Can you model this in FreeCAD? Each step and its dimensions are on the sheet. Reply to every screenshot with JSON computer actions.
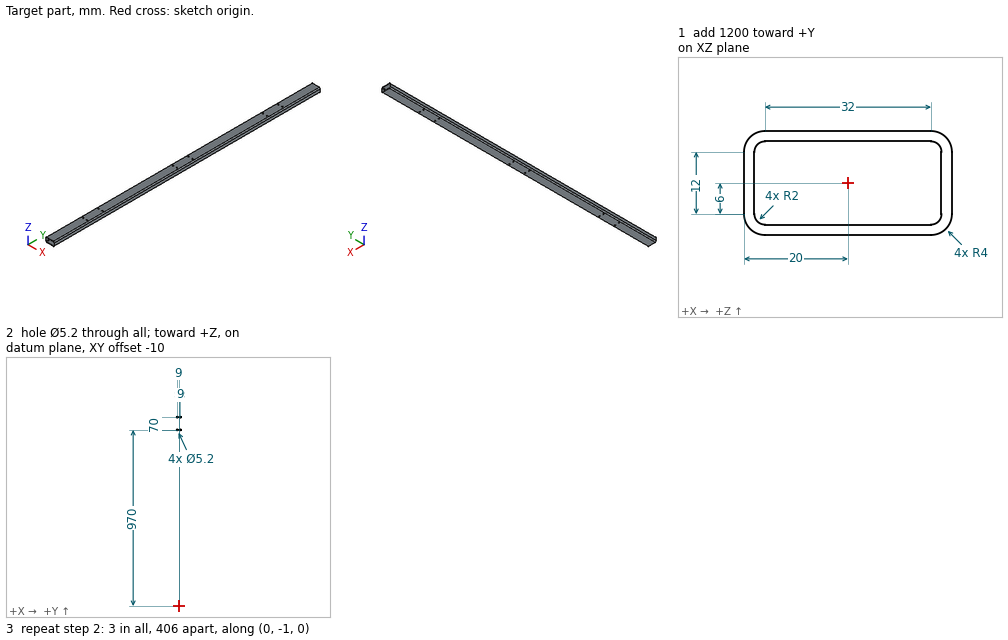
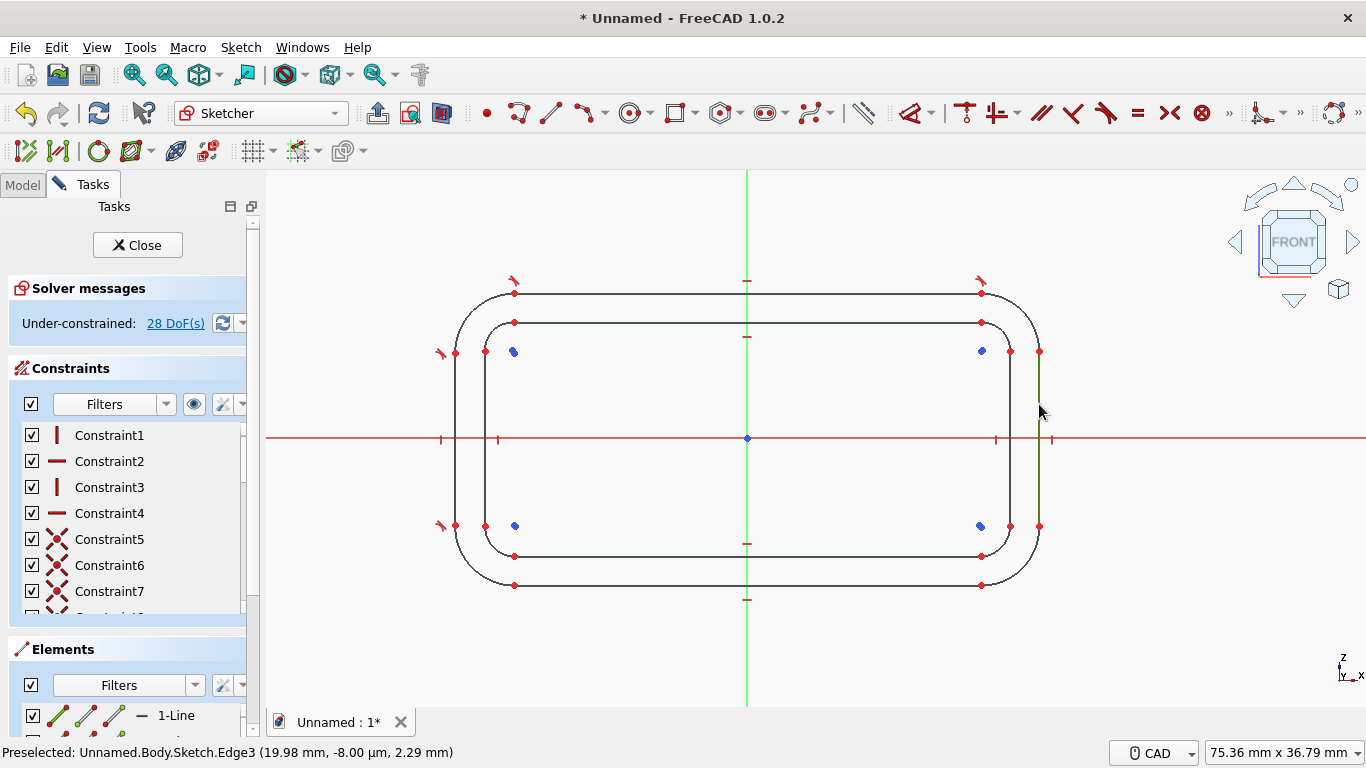
{"action": "left_click", "coordinate": [1033, 325]}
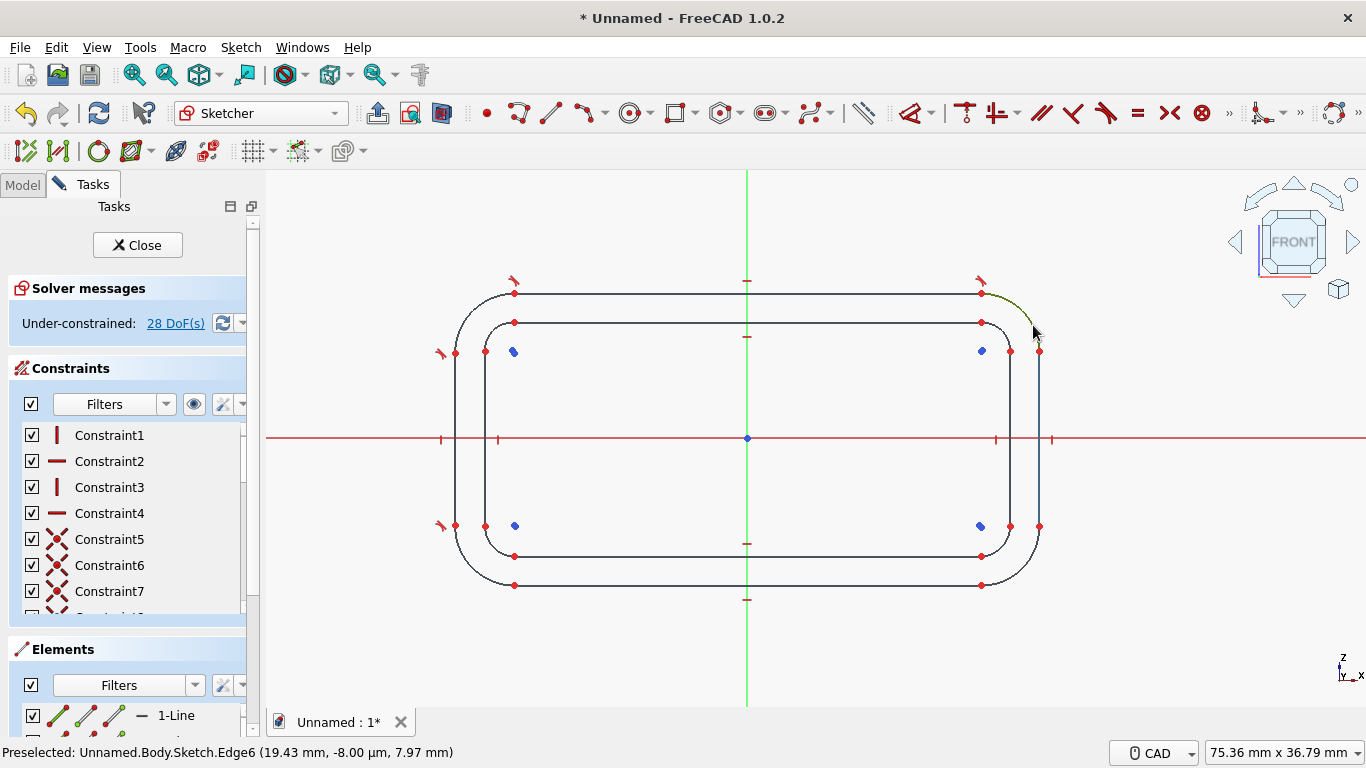
{"action": "left_click", "coordinate": [1106, 114]}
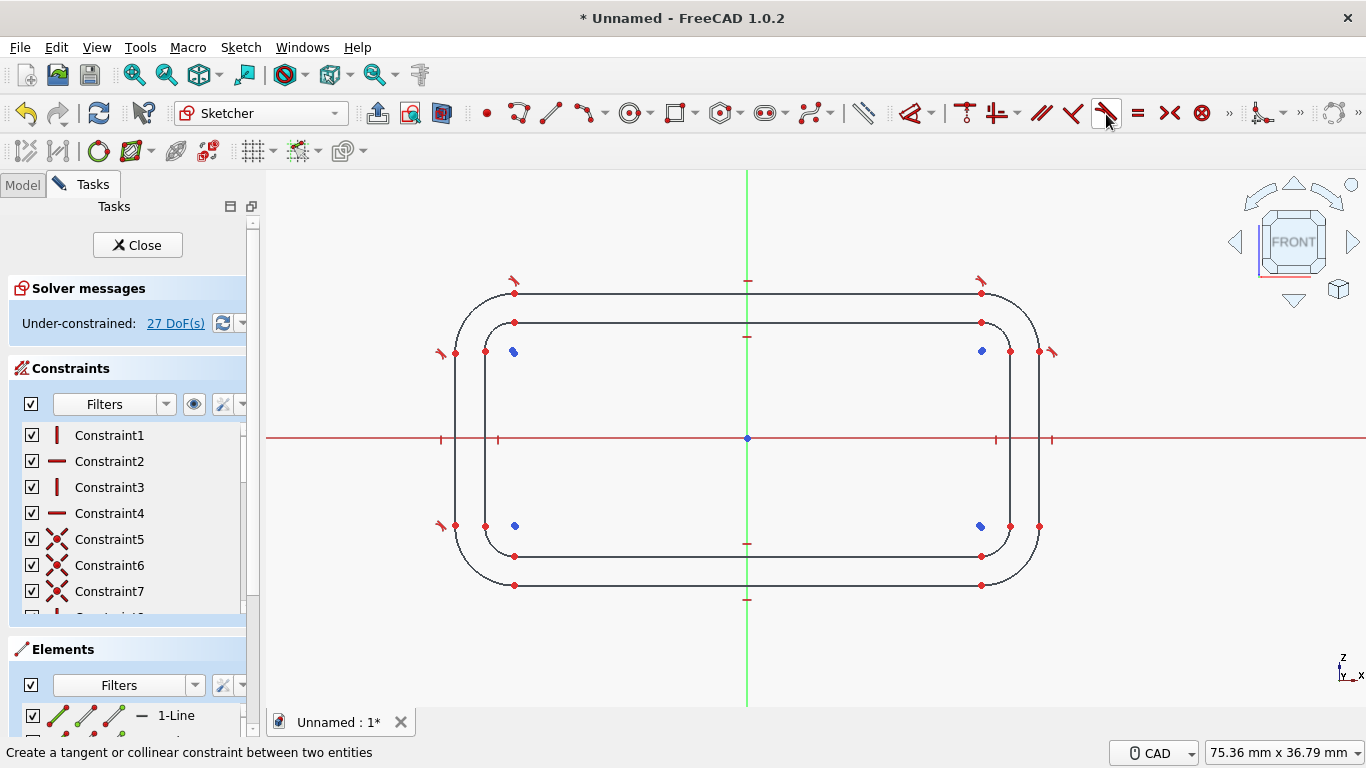
{"action": "left_click", "coordinate": [1039, 404]}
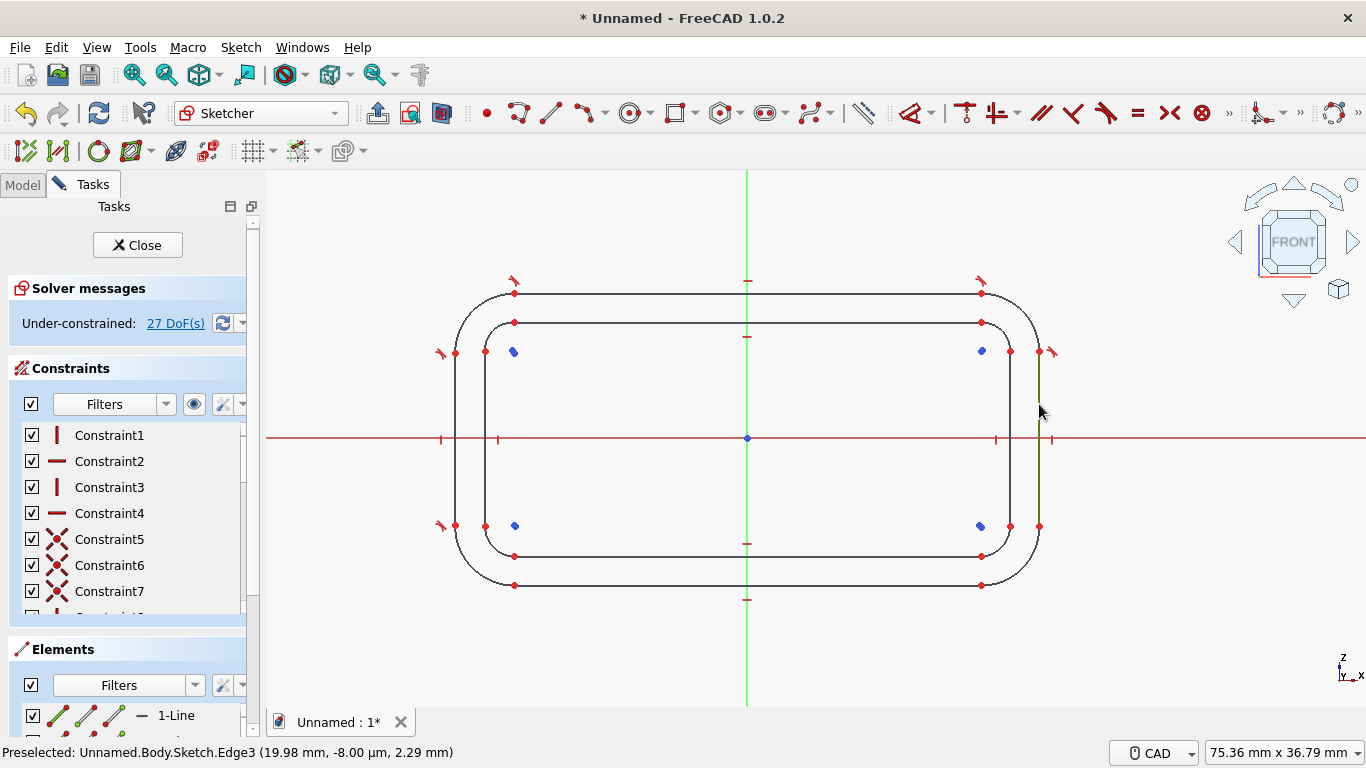
{"action": "left_click", "coordinate": [1008, 579]}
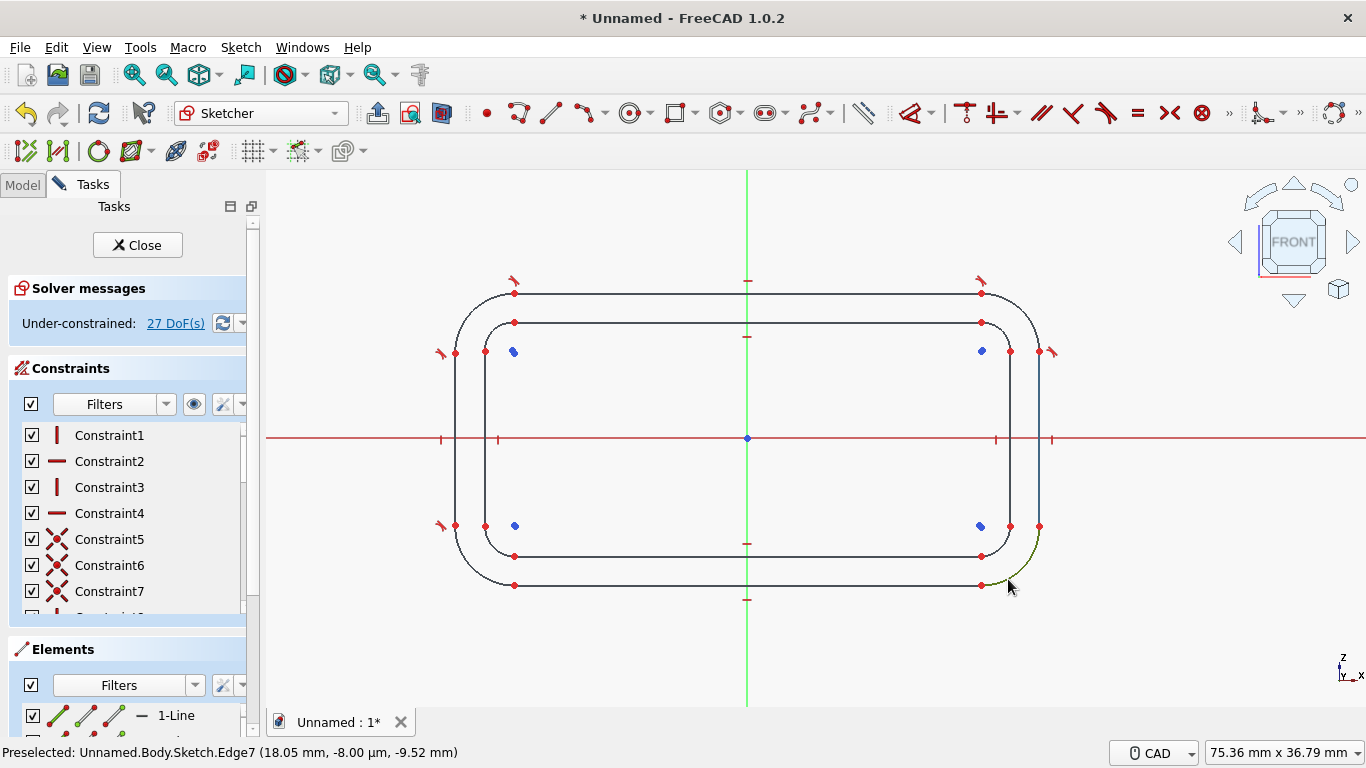
{"action": "key", "text": "t"}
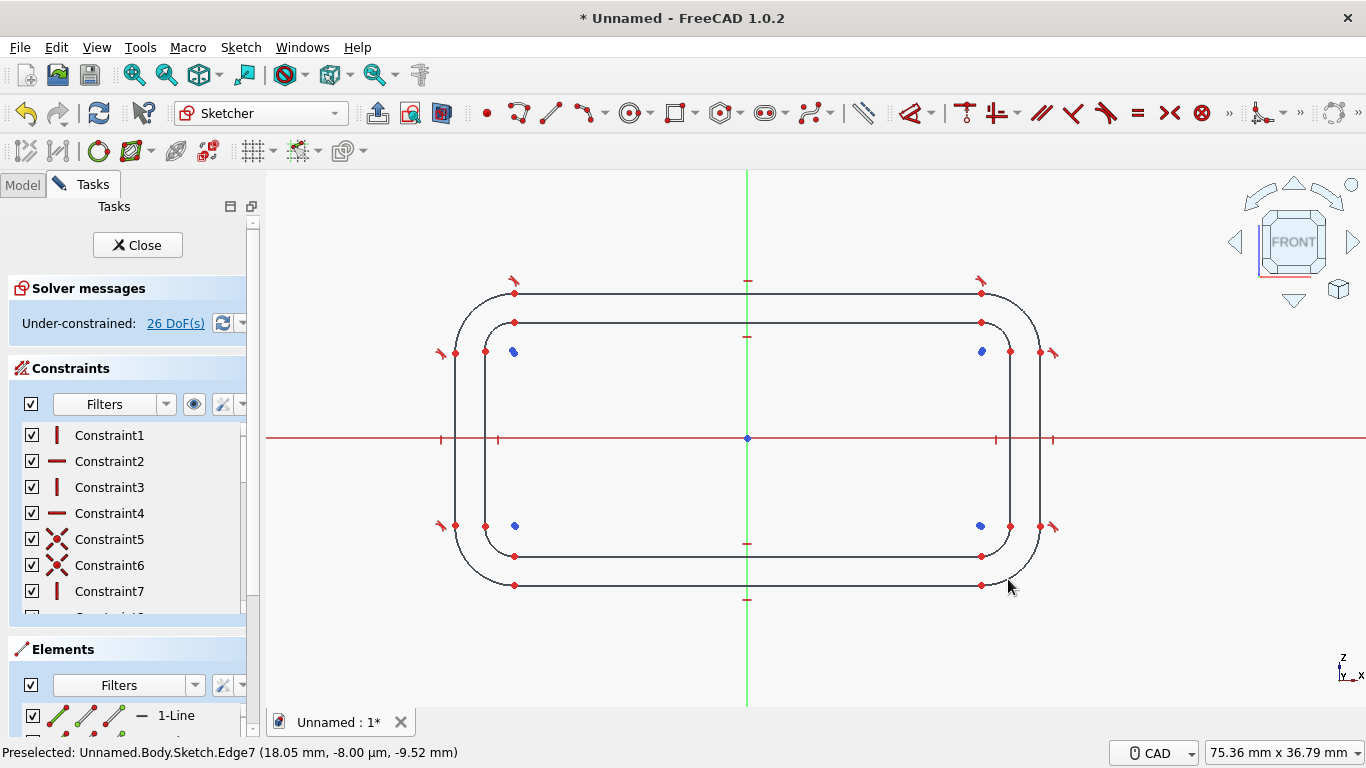
{"action": "left_click", "coordinate": [841, 586]}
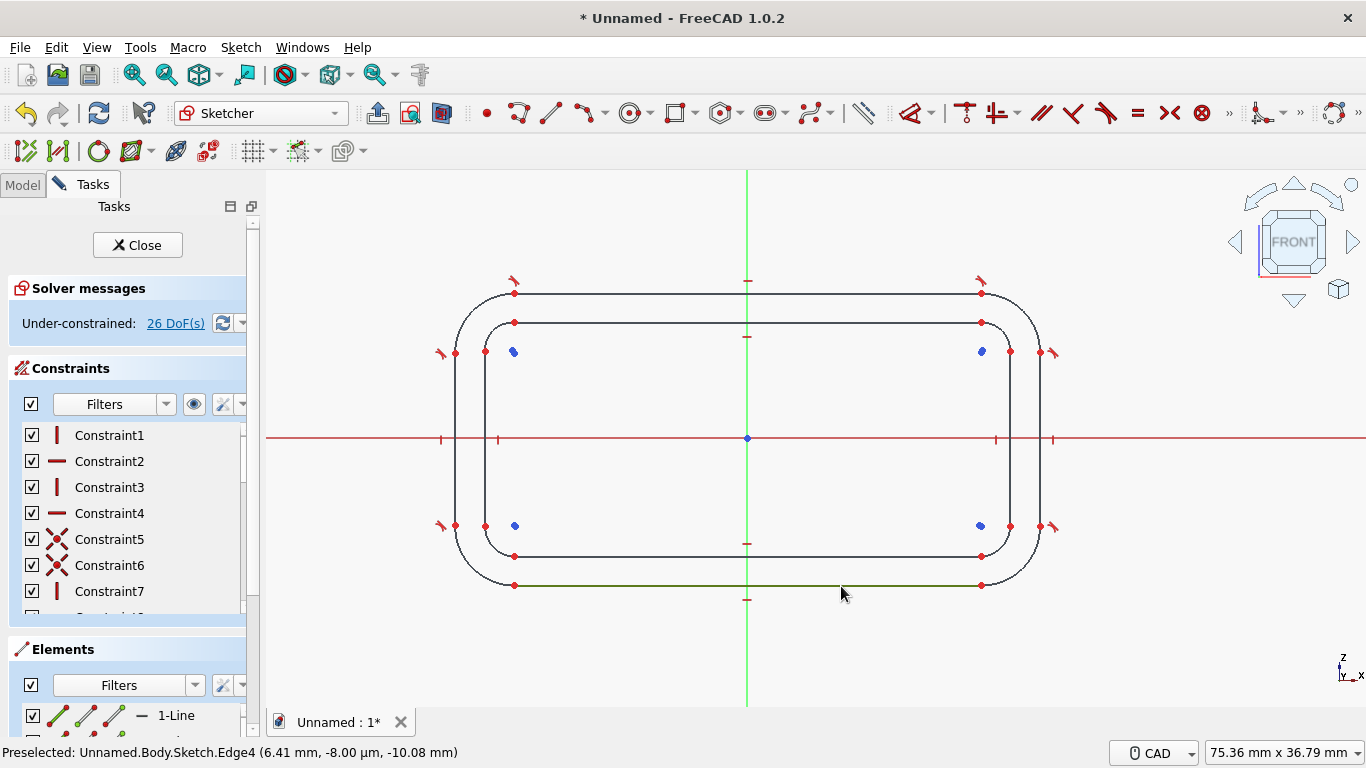
{"action": "left_click", "coordinate": [1008, 579]}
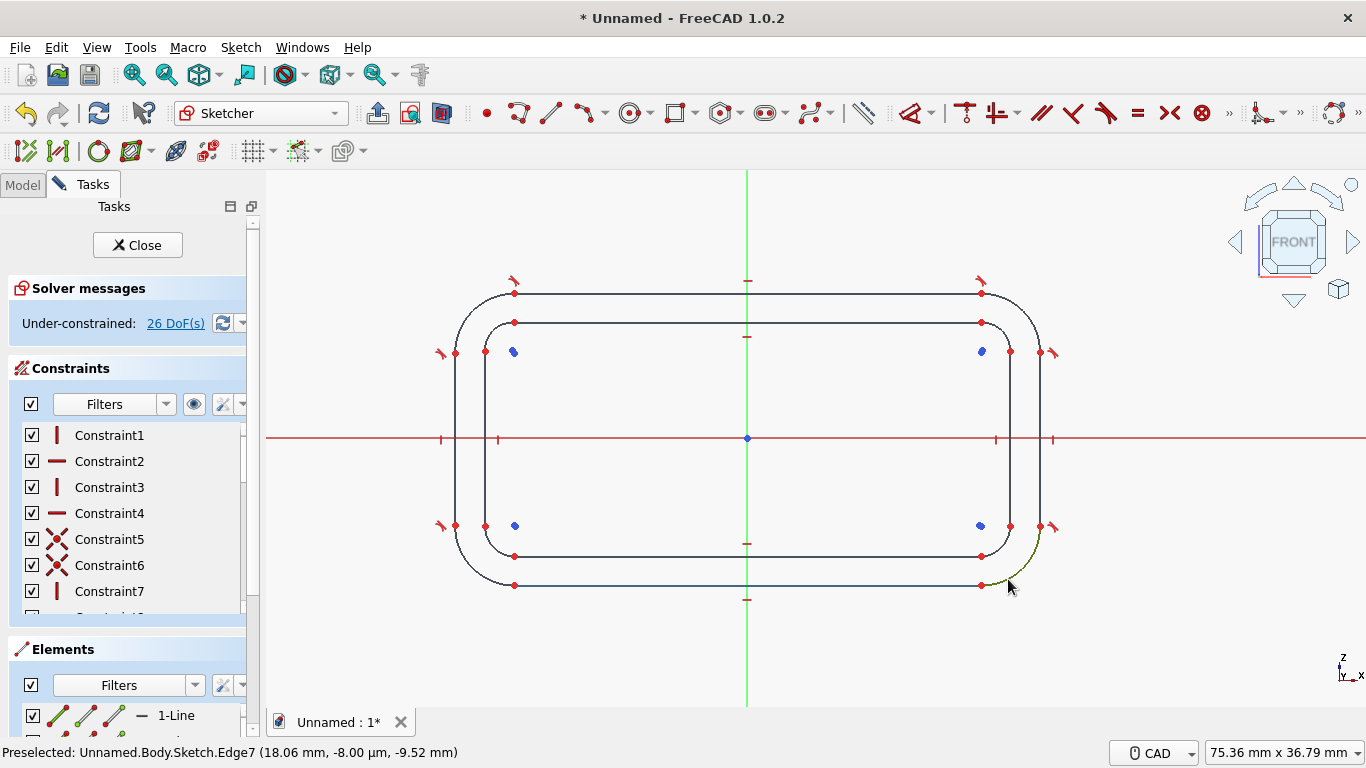
{"action": "left_click", "coordinate": [1106, 114]}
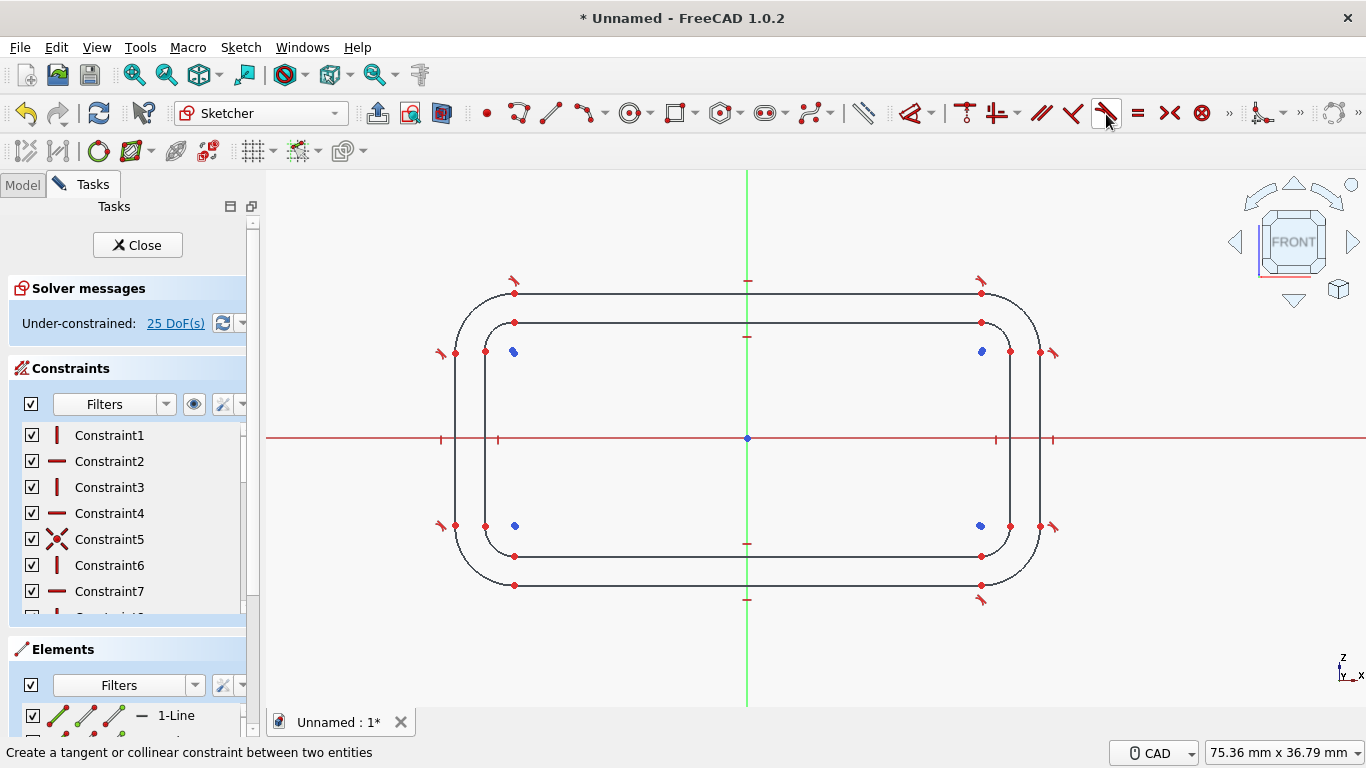
{"action": "left_click", "coordinate": [841, 586]}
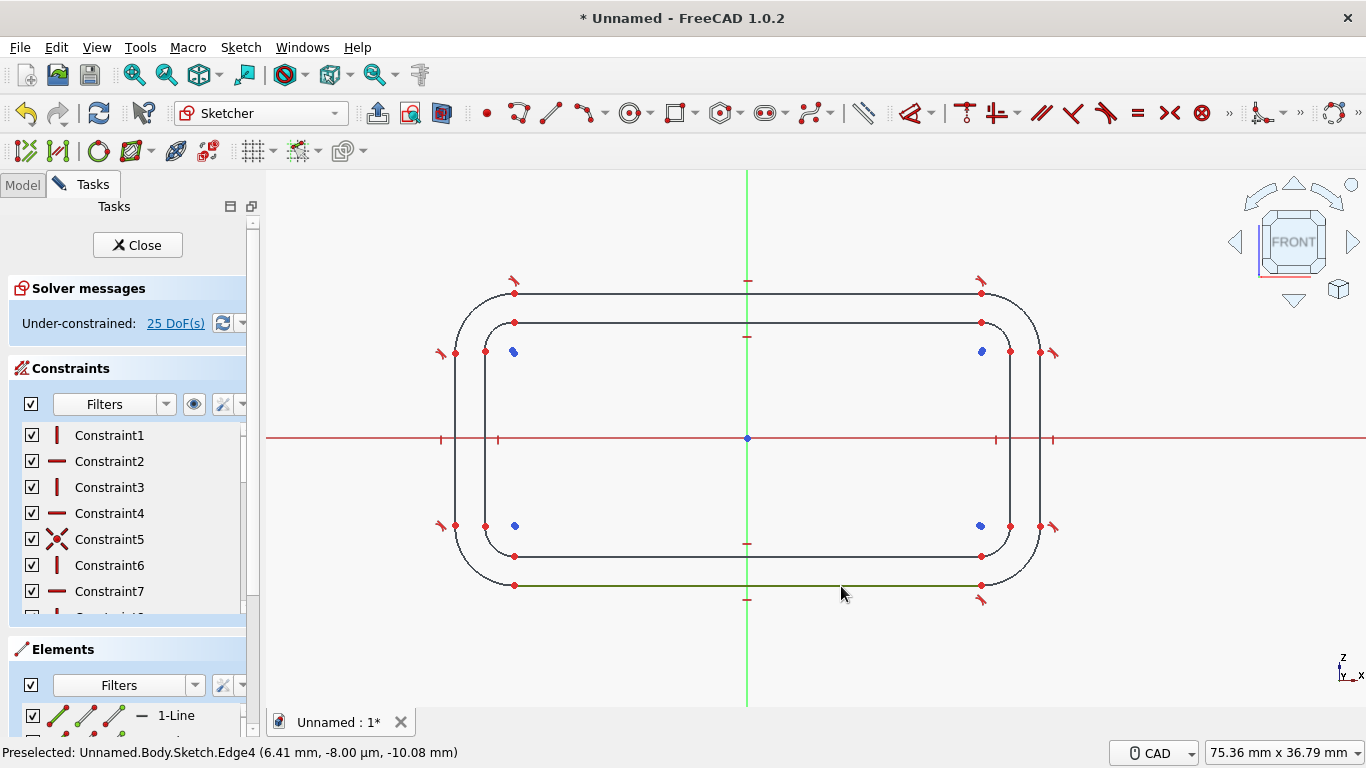
{"action": "left_click", "coordinate": [462, 553]}